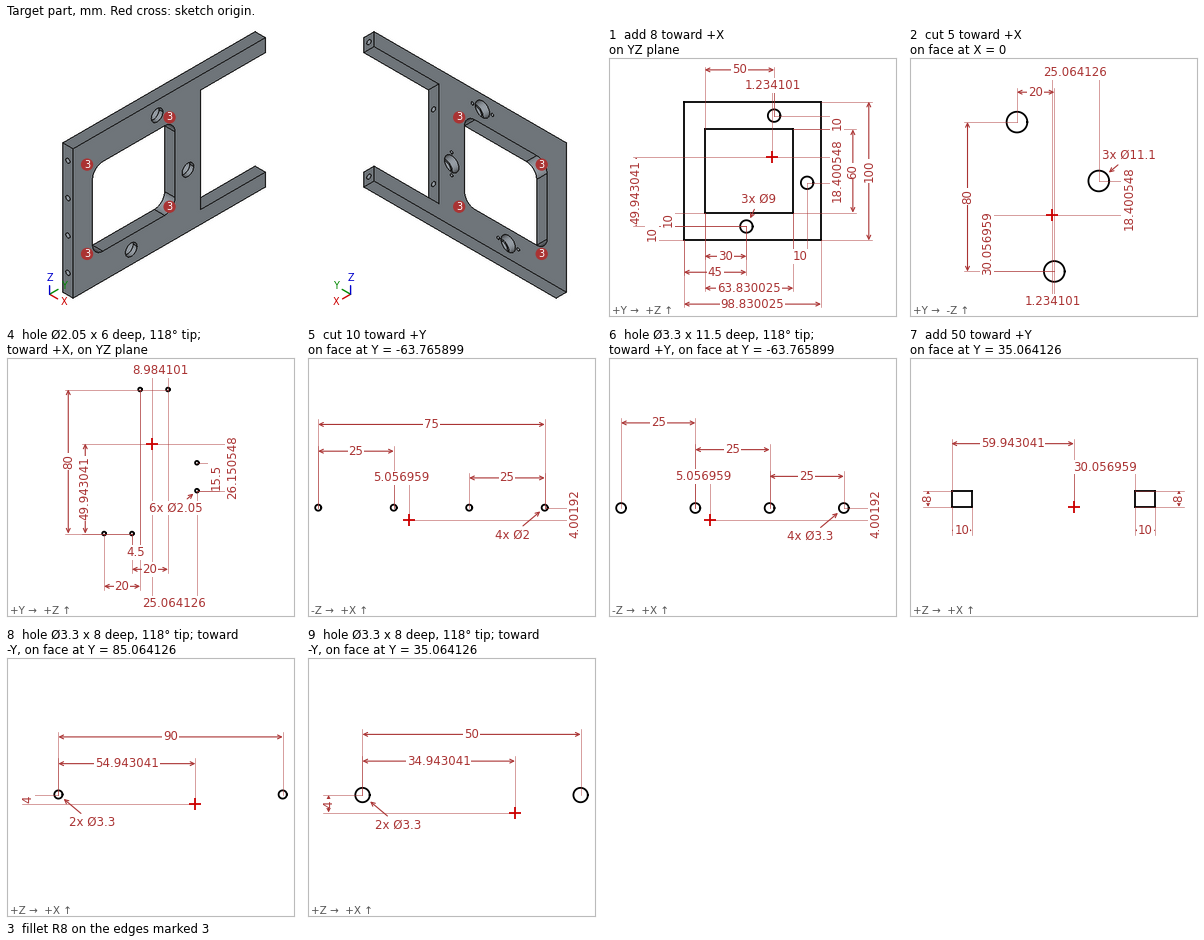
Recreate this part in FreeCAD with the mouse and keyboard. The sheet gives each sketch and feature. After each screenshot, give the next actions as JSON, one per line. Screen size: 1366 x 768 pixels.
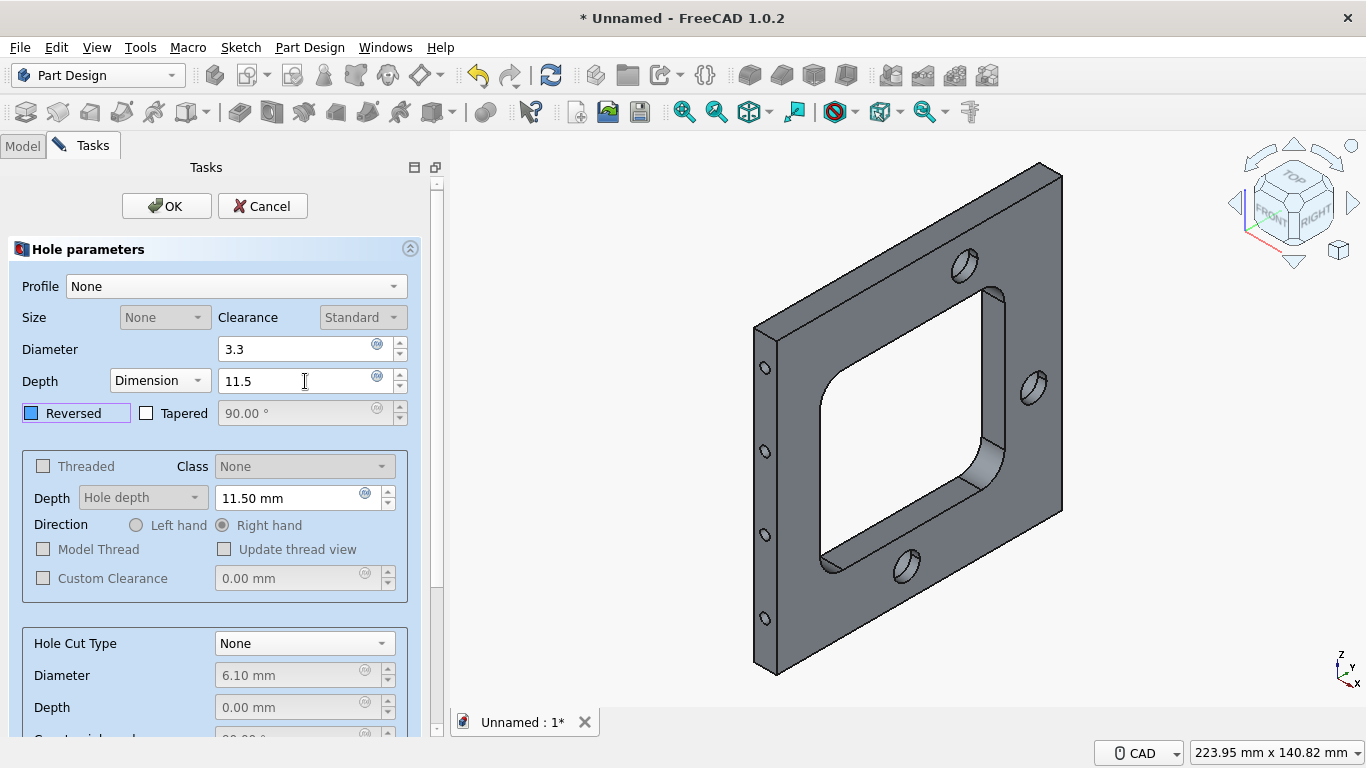
{"action": "left_click", "coordinate": [167, 206]}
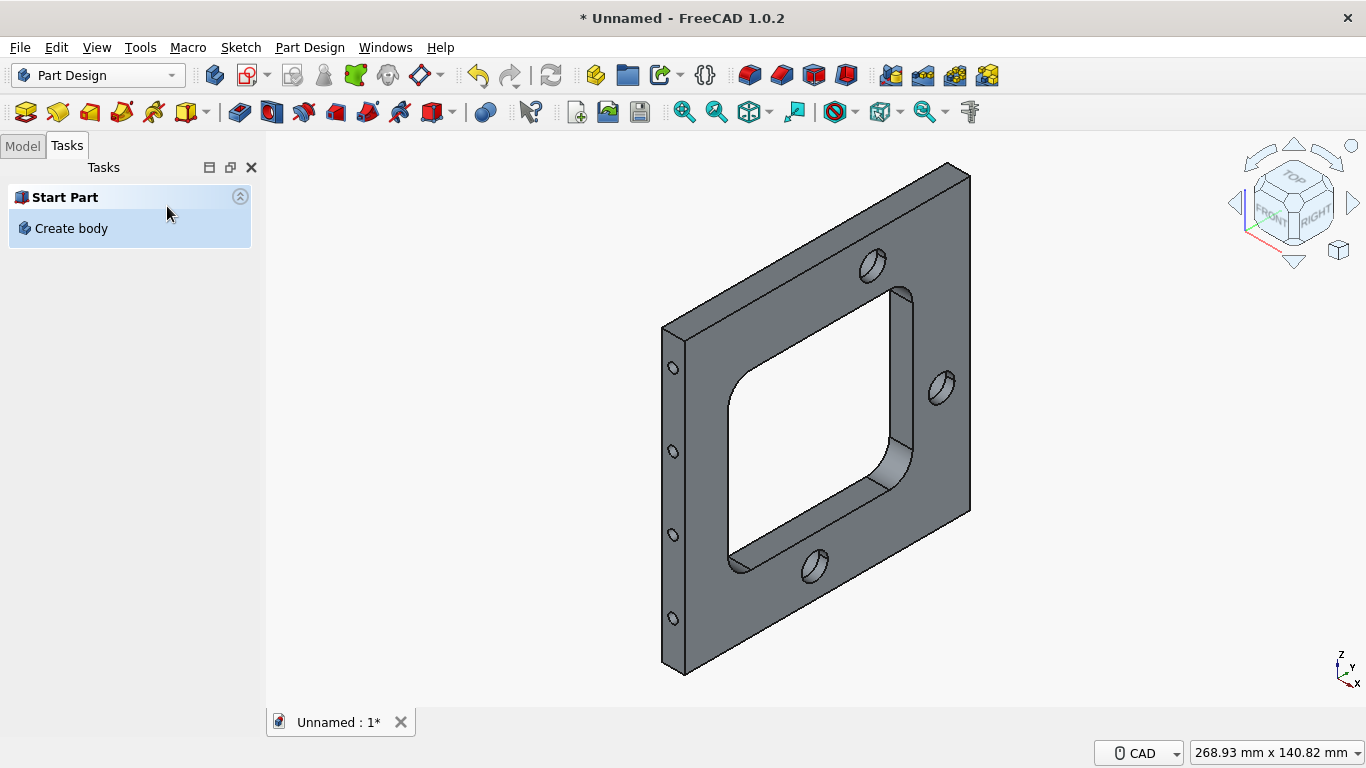
{"action": "key", "text": "4"}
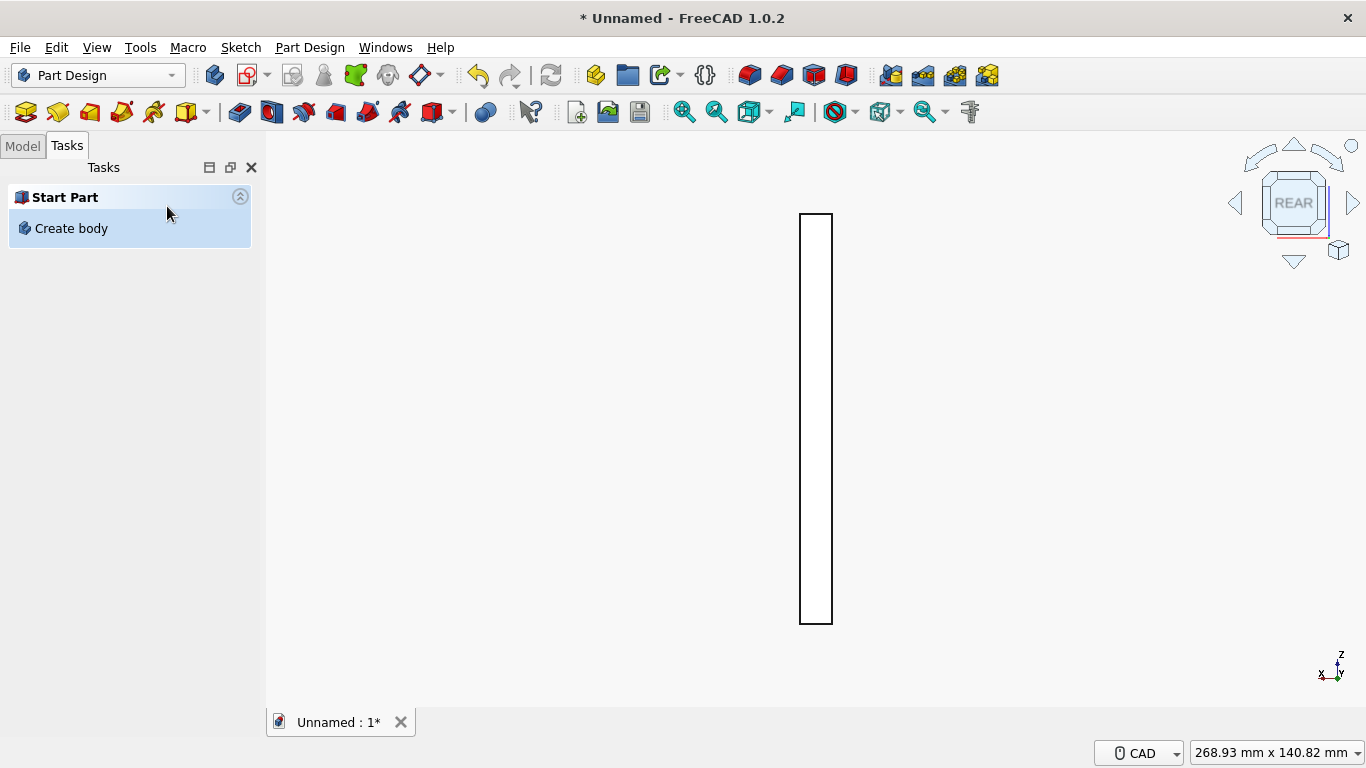
{"action": "left_click", "coordinate": [816, 535]}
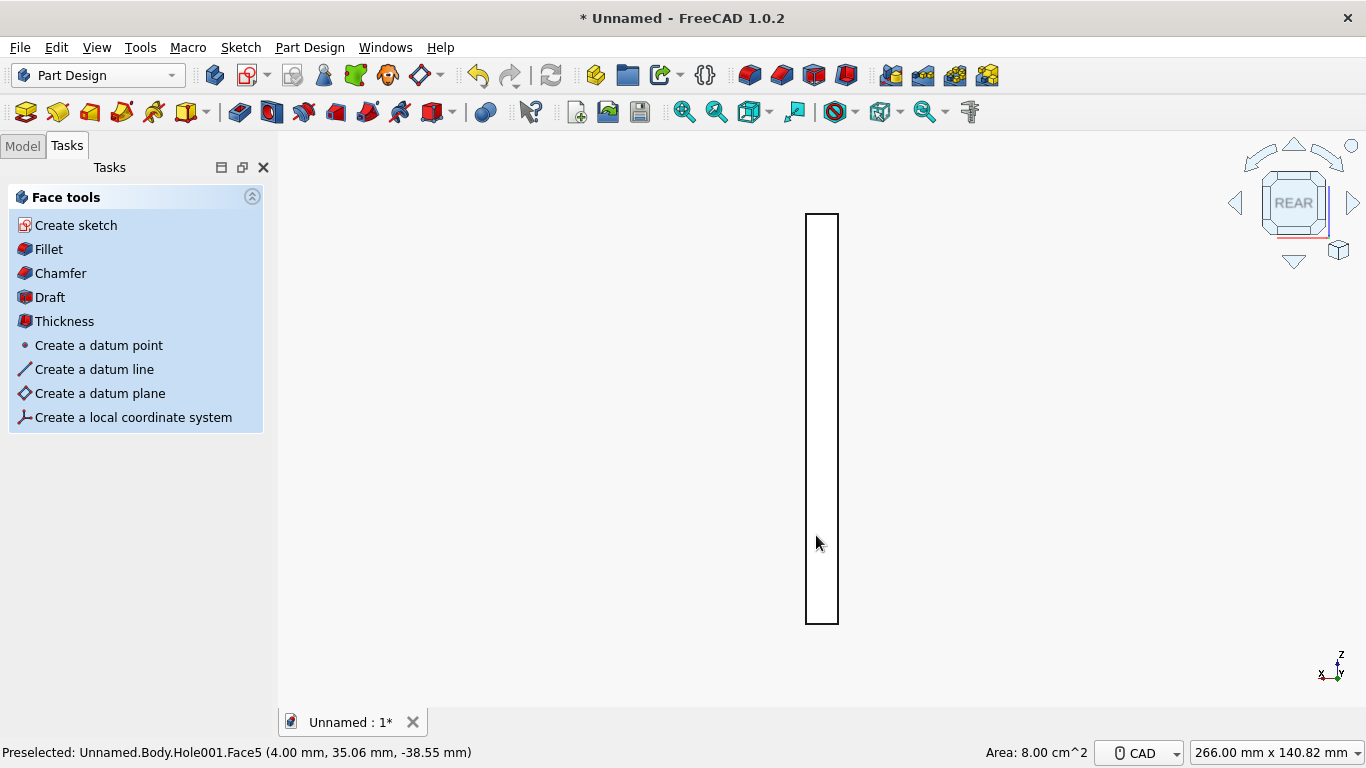
{"action": "left_click", "coordinate": [248, 76]}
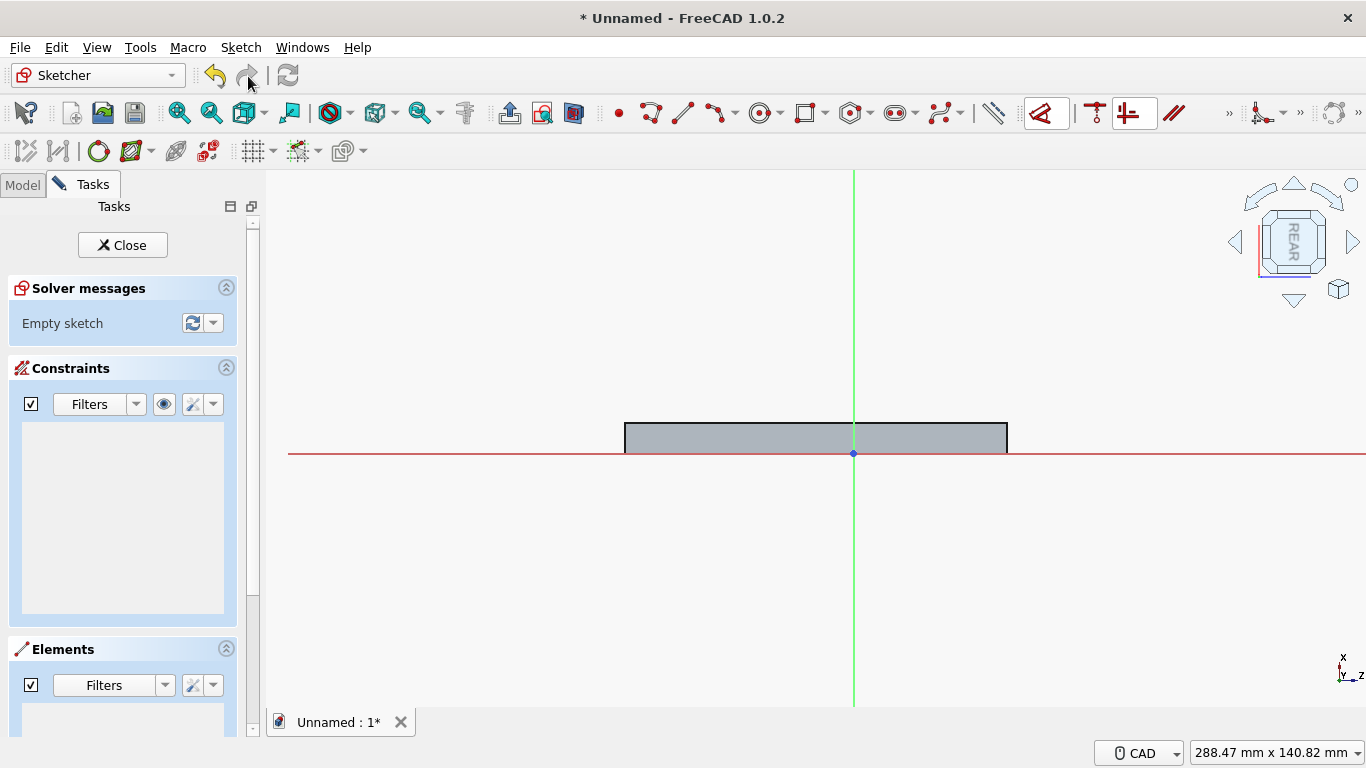
{"action": "scroll", "coordinate": [899, 439], "scroll_direction": "up", "scroll_amount": 3}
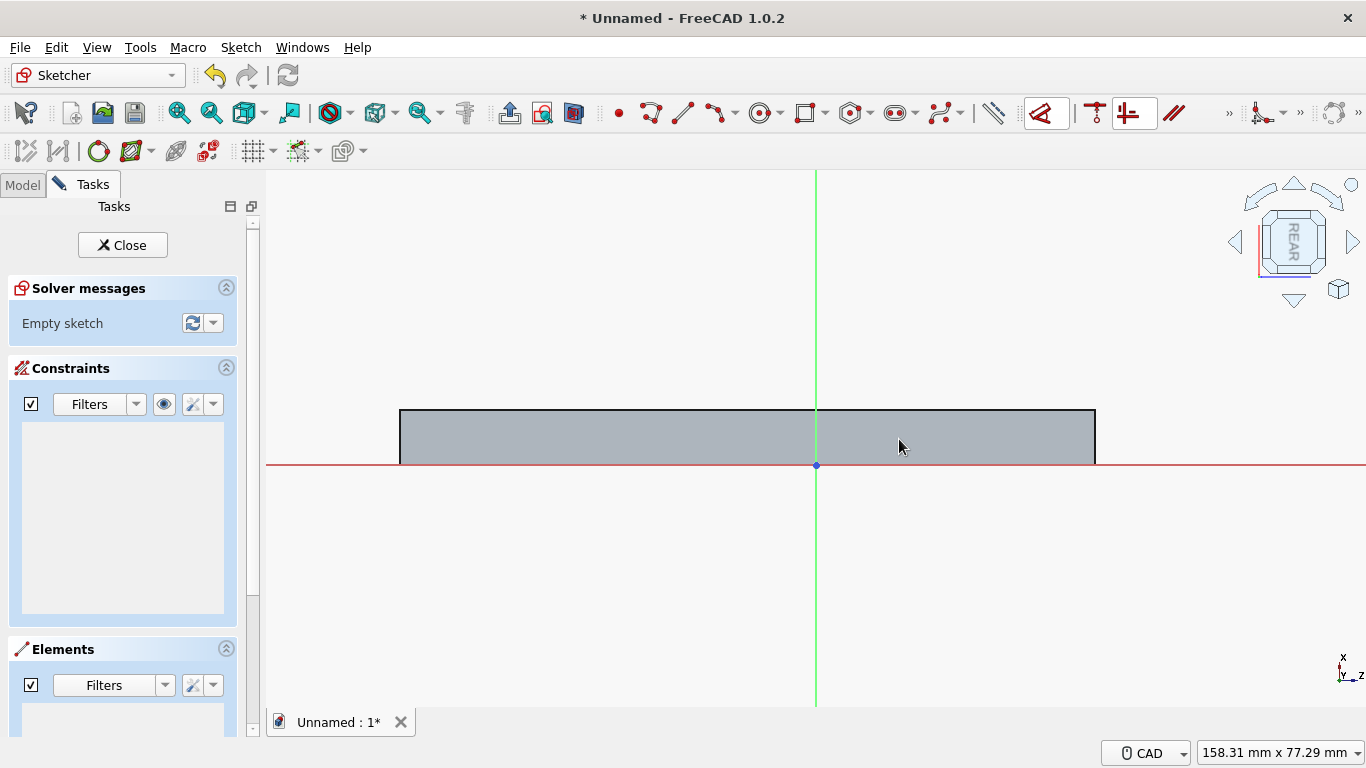
{"action": "left_click", "coordinate": [806, 114]}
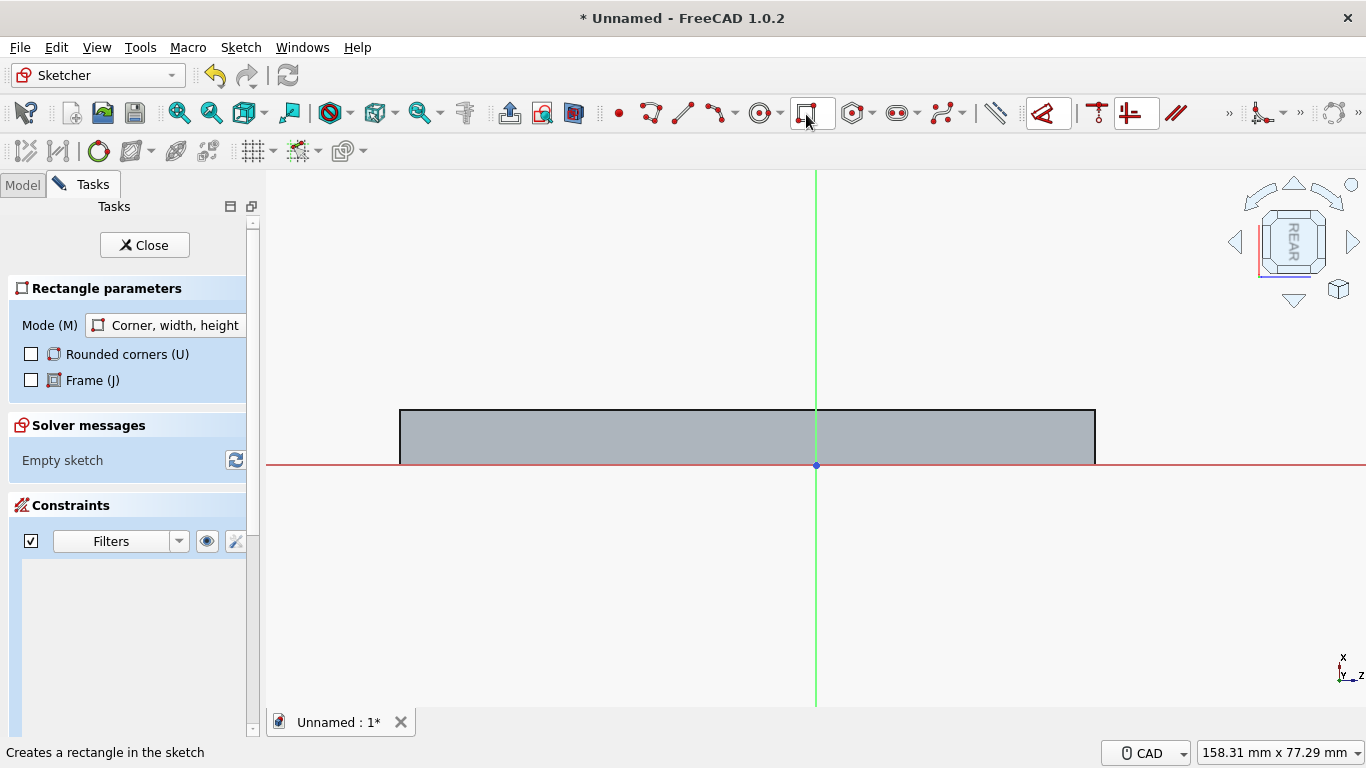
{"action": "left_click", "coordinate": [400, 410]}
{"action": "left_click", "coordinate": [469, 465]}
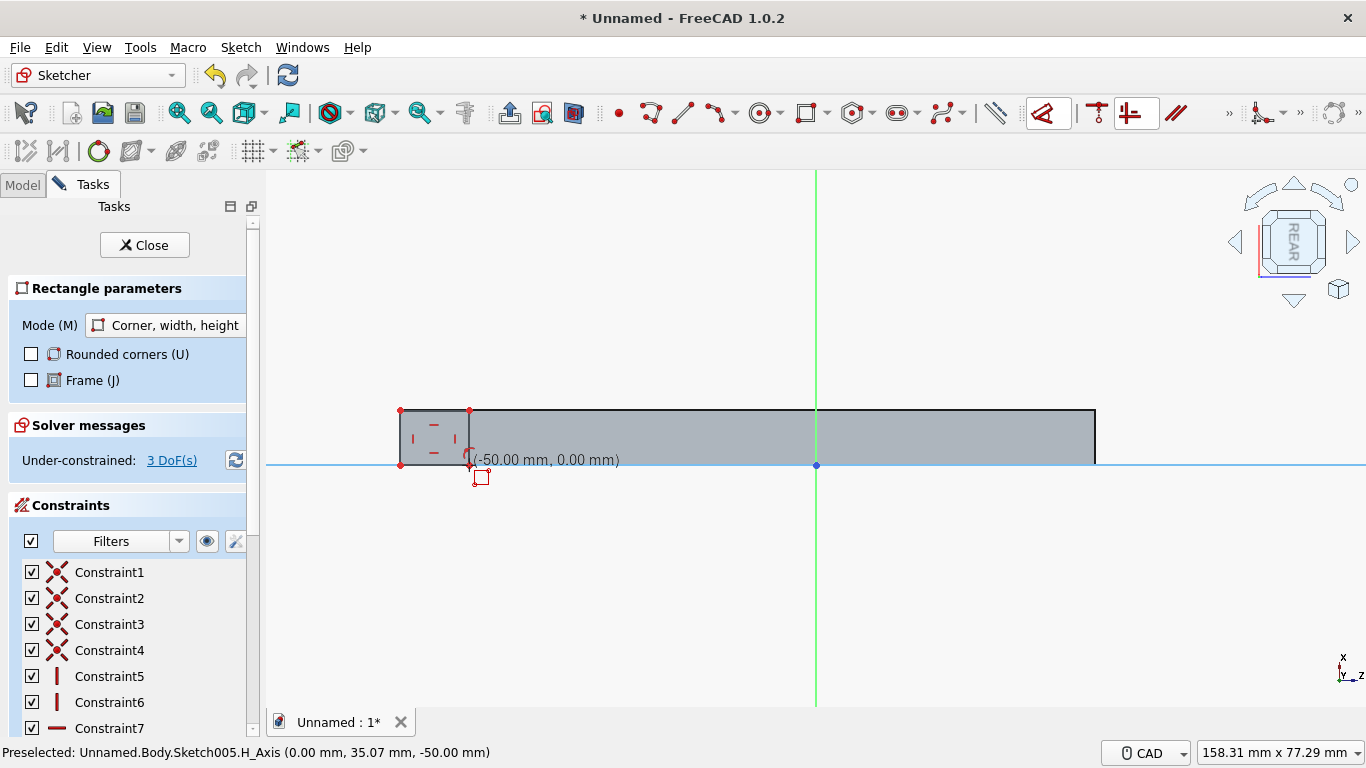
{"action": "left_click", "coordinate": [1025, 410]}
{"action": "left_click", "coordinate": [1095, 465]}
{"action": "key", "text": "Escape"}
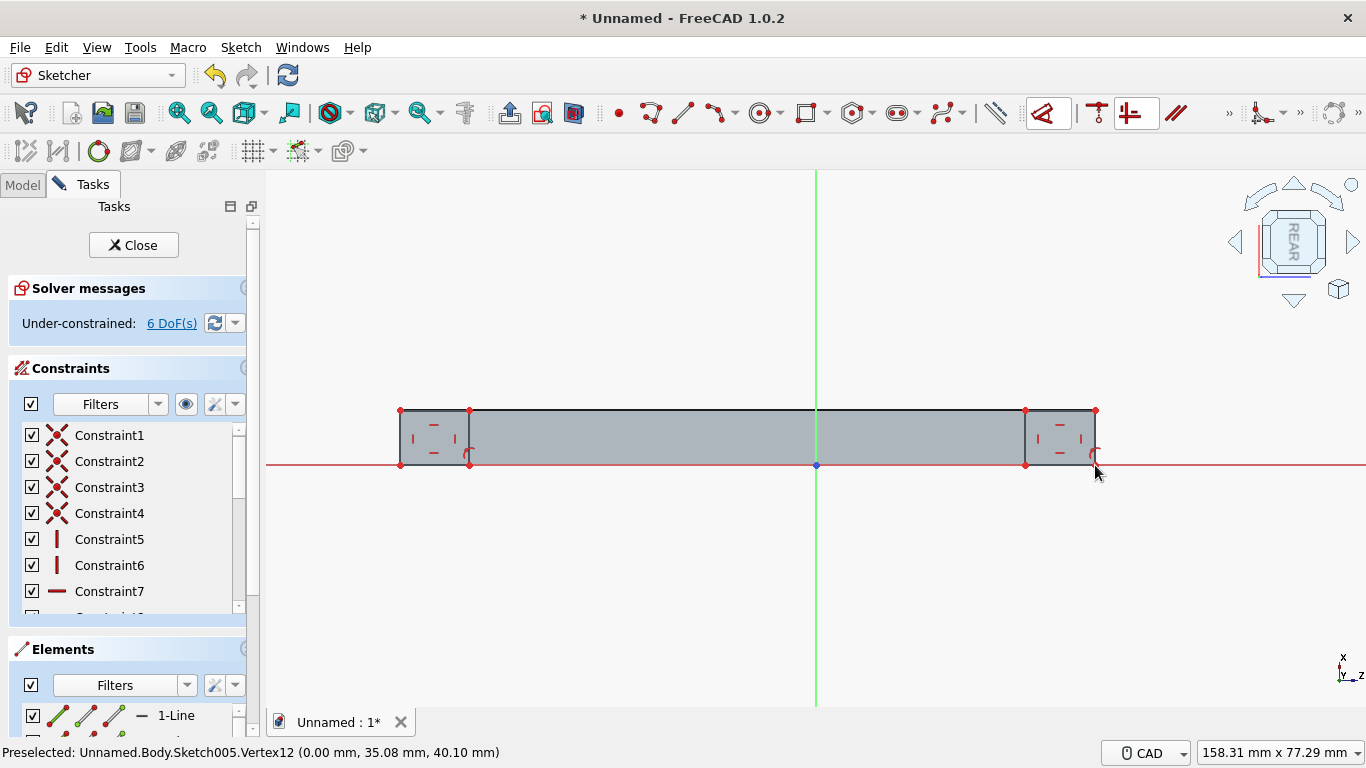
{"action": "left_click", "coordinate": [400, 427]}